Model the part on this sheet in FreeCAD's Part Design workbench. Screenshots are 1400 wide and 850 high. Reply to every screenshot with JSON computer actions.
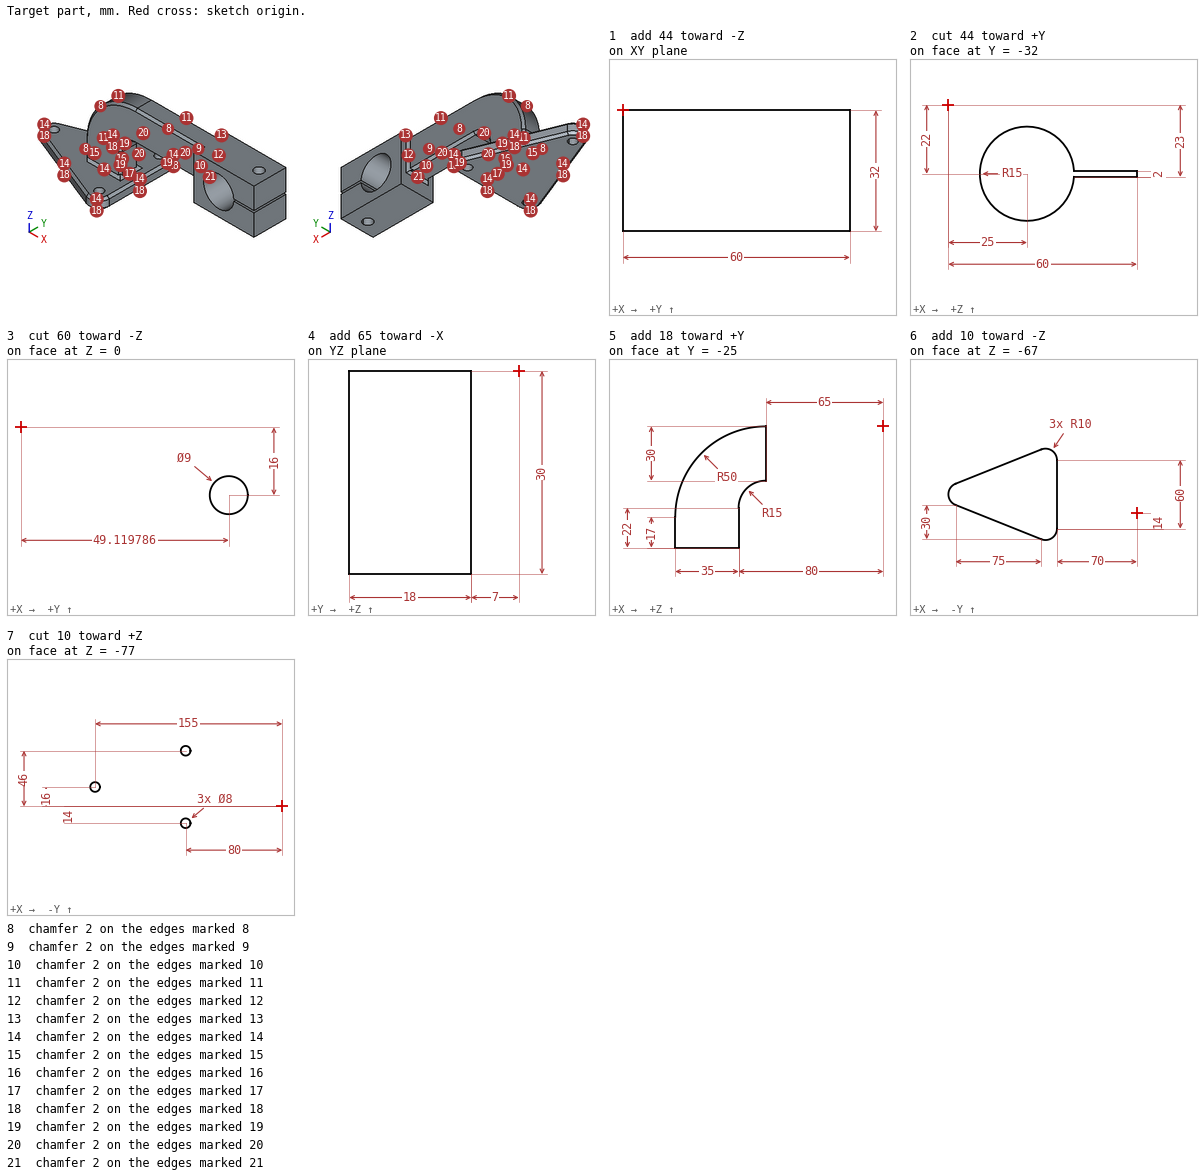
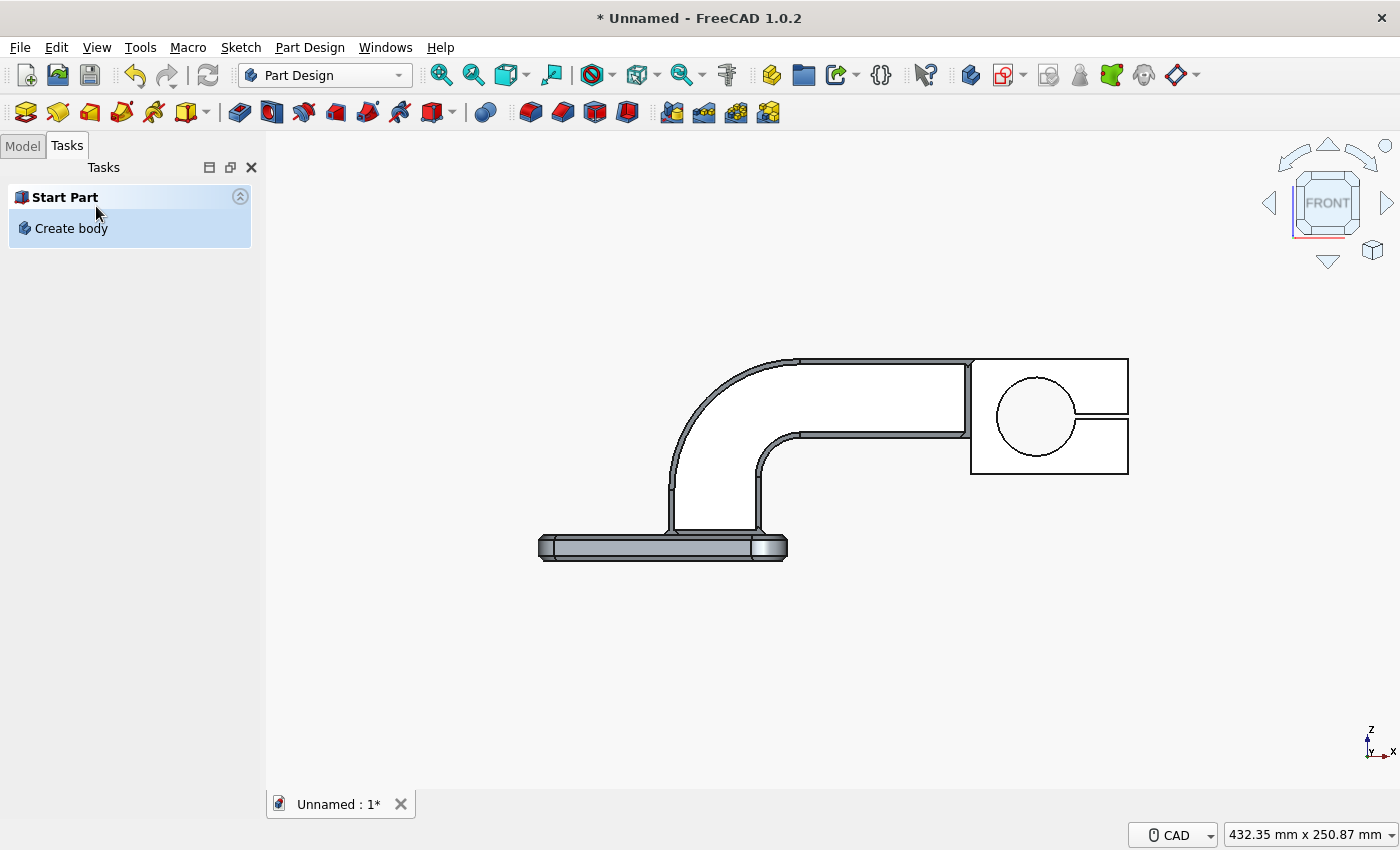
{"action": "key", "text": "3"}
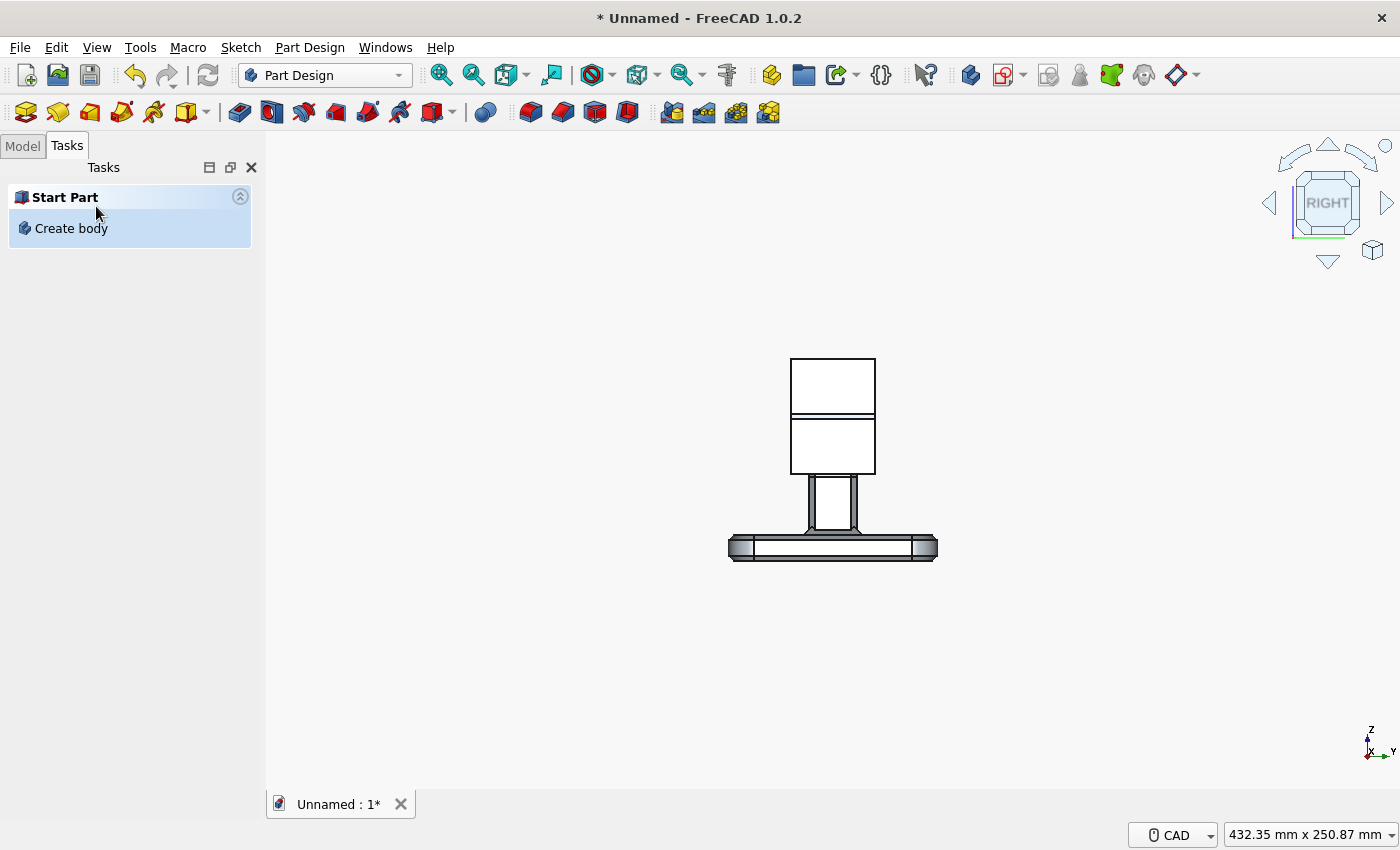
{"action": "left_click", "coordinate": [442, 76]}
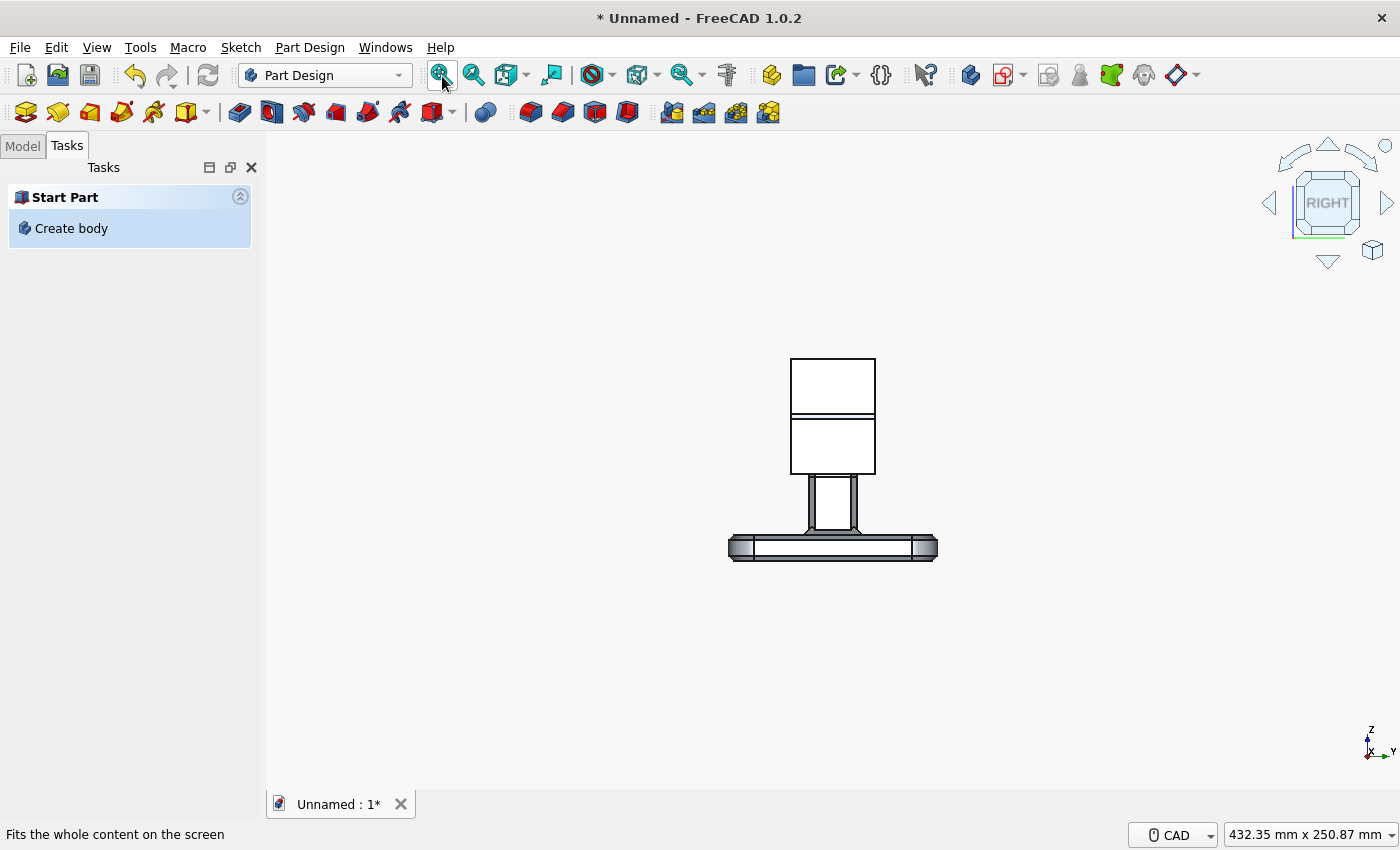
{"action": "key", "text": "5"}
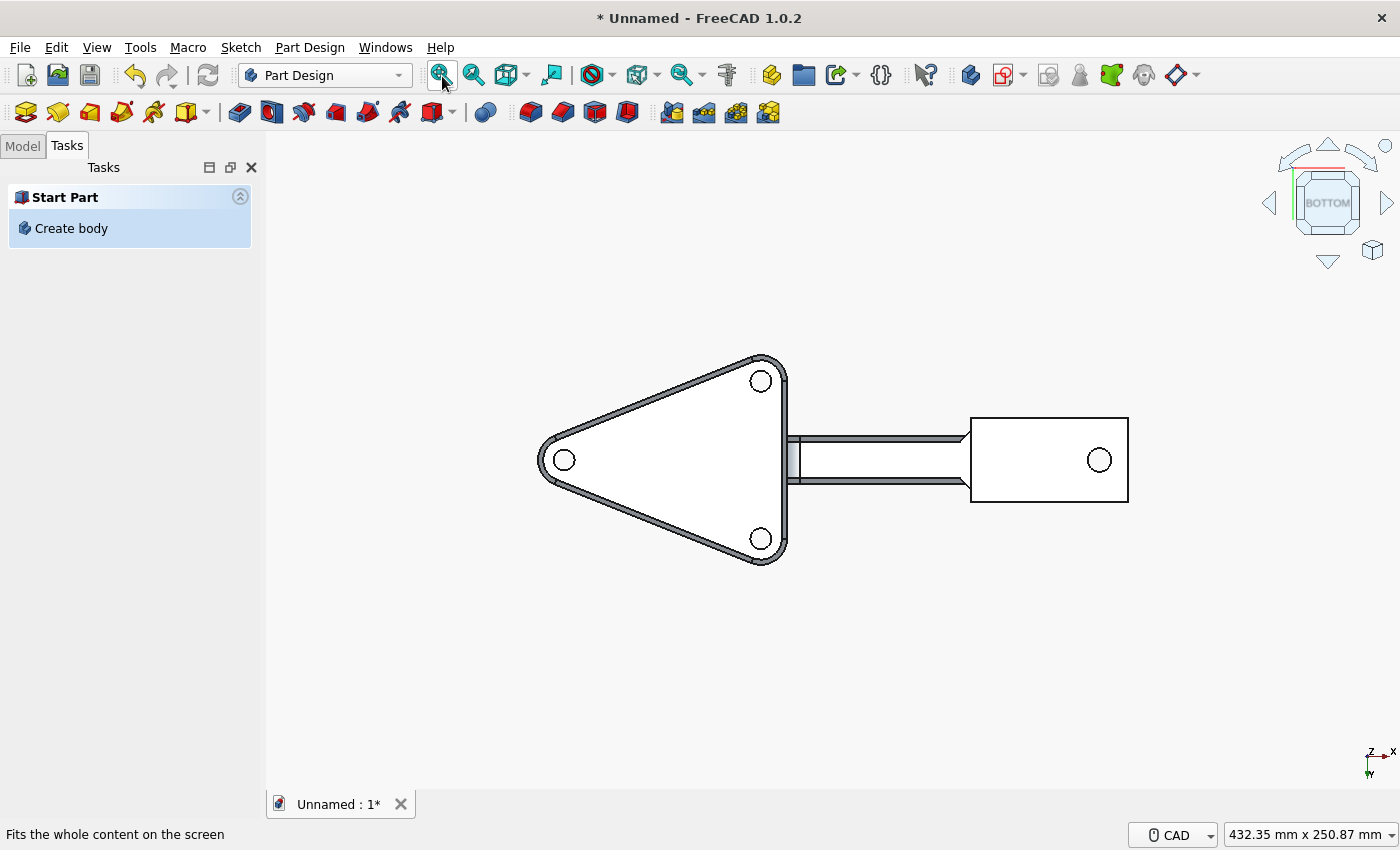
{"action": "key", "text": "4"}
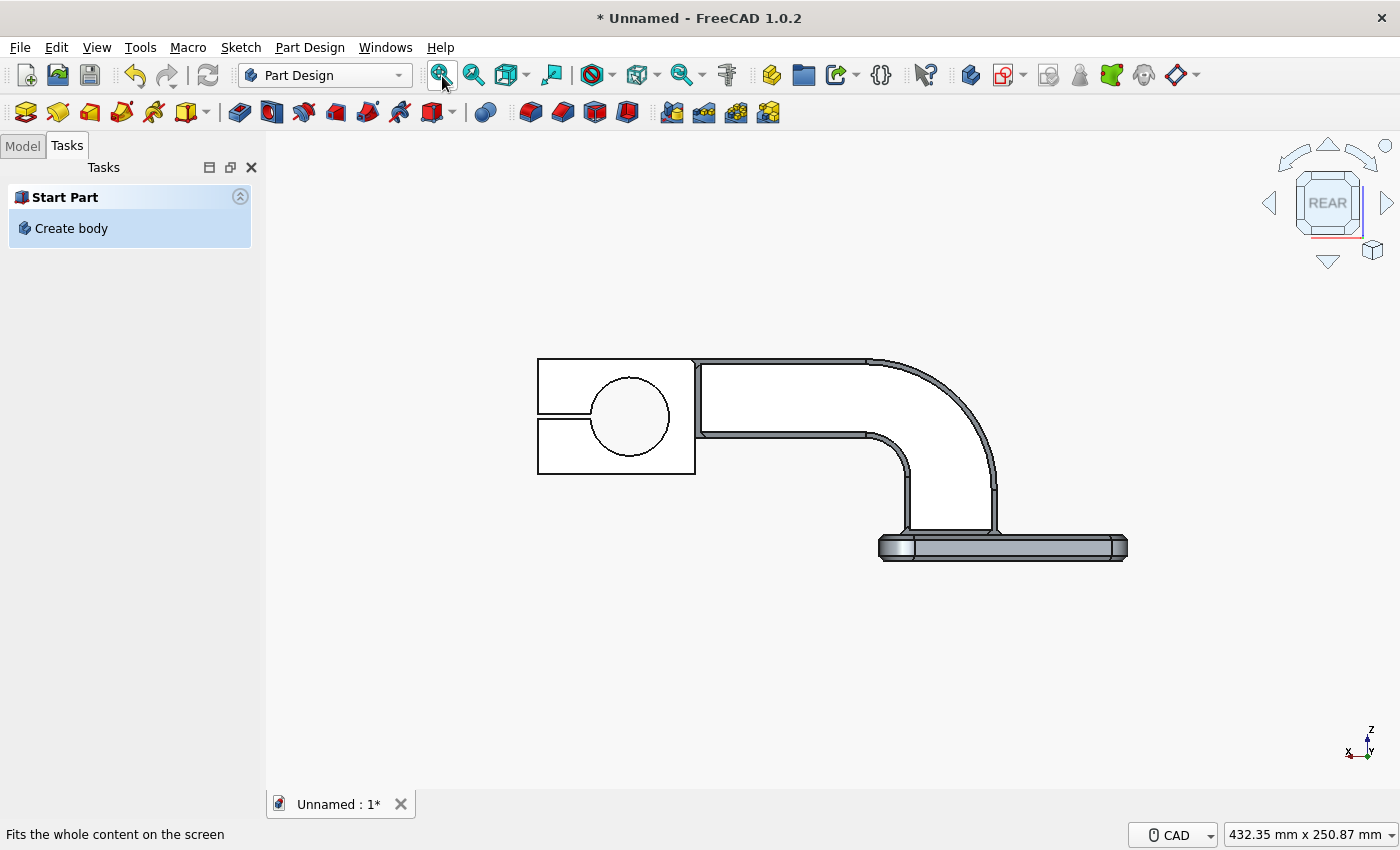
{"action": "key", "text": "6"}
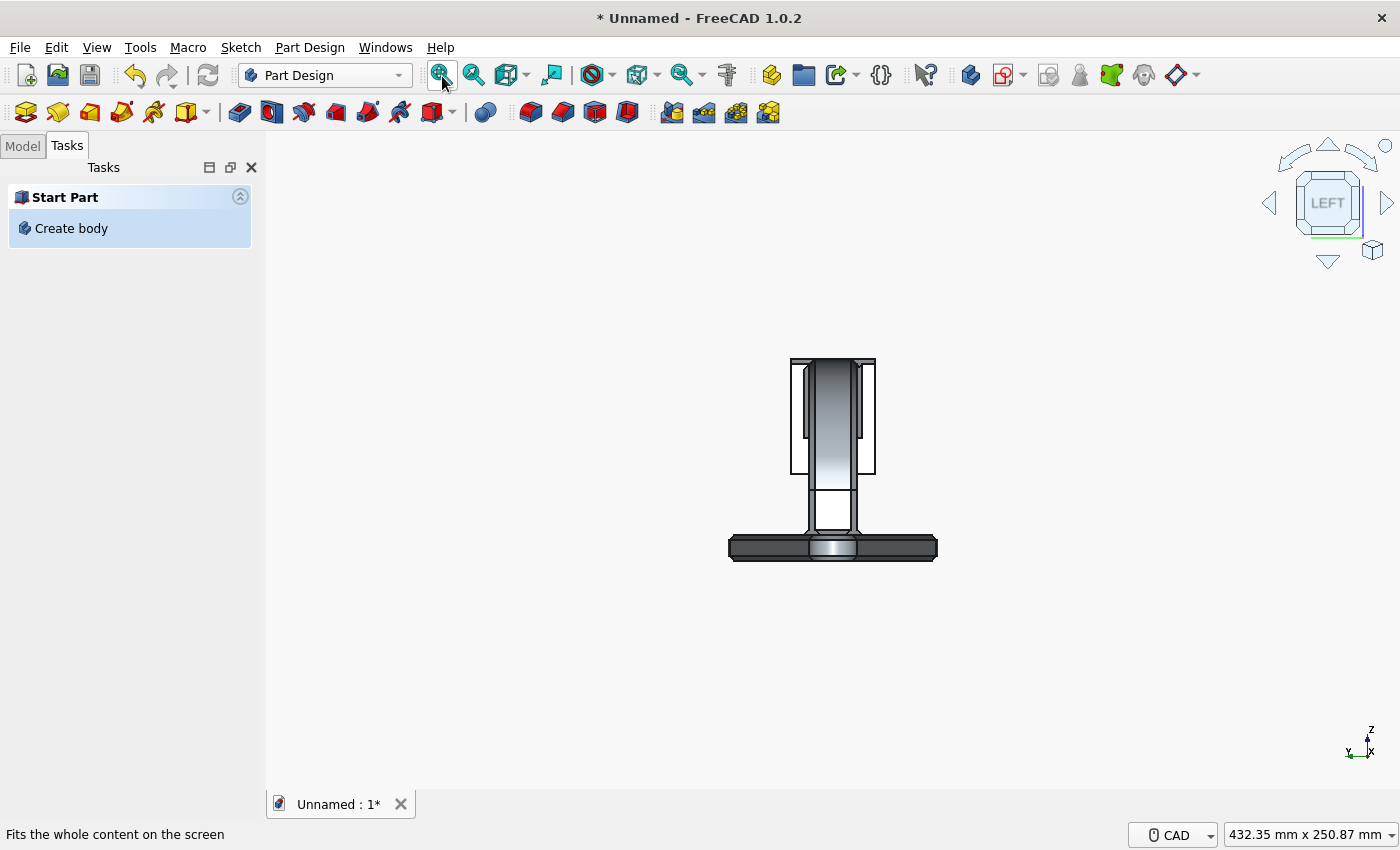
{"action": "left_click", "coordinate": [442, 76]}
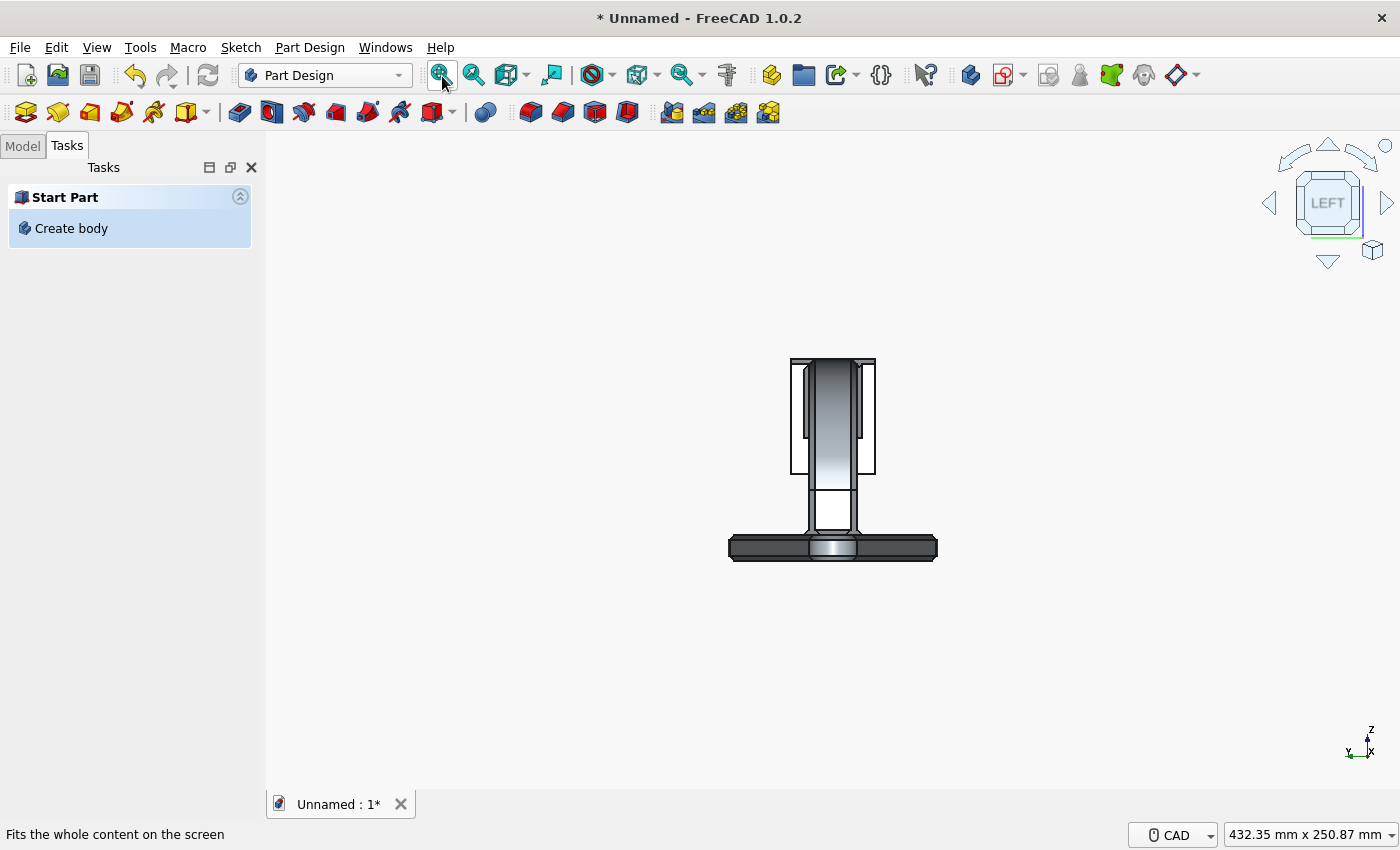
{"action": "key", "text": "v 3"}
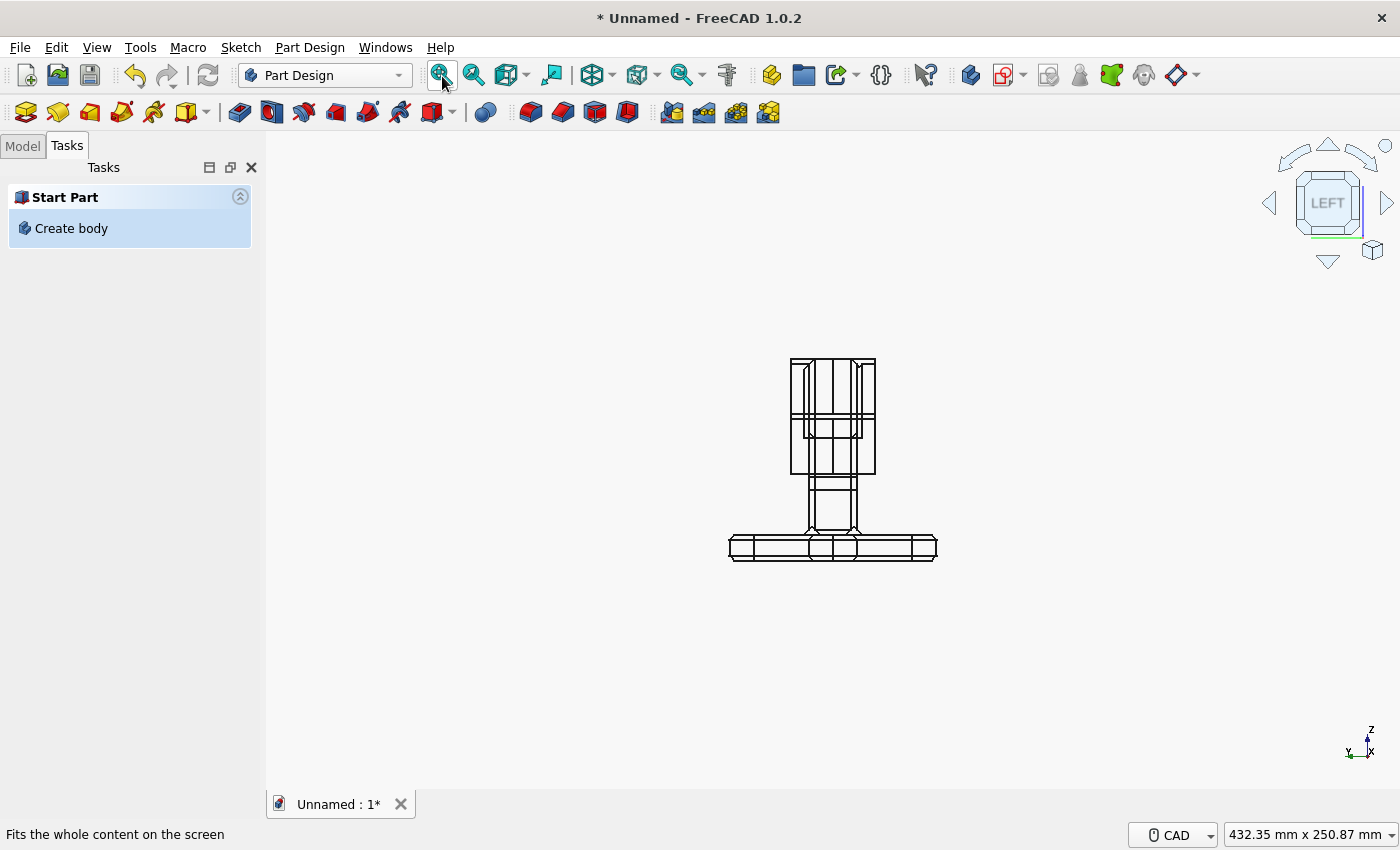
{"action": "key", "text": "0"}